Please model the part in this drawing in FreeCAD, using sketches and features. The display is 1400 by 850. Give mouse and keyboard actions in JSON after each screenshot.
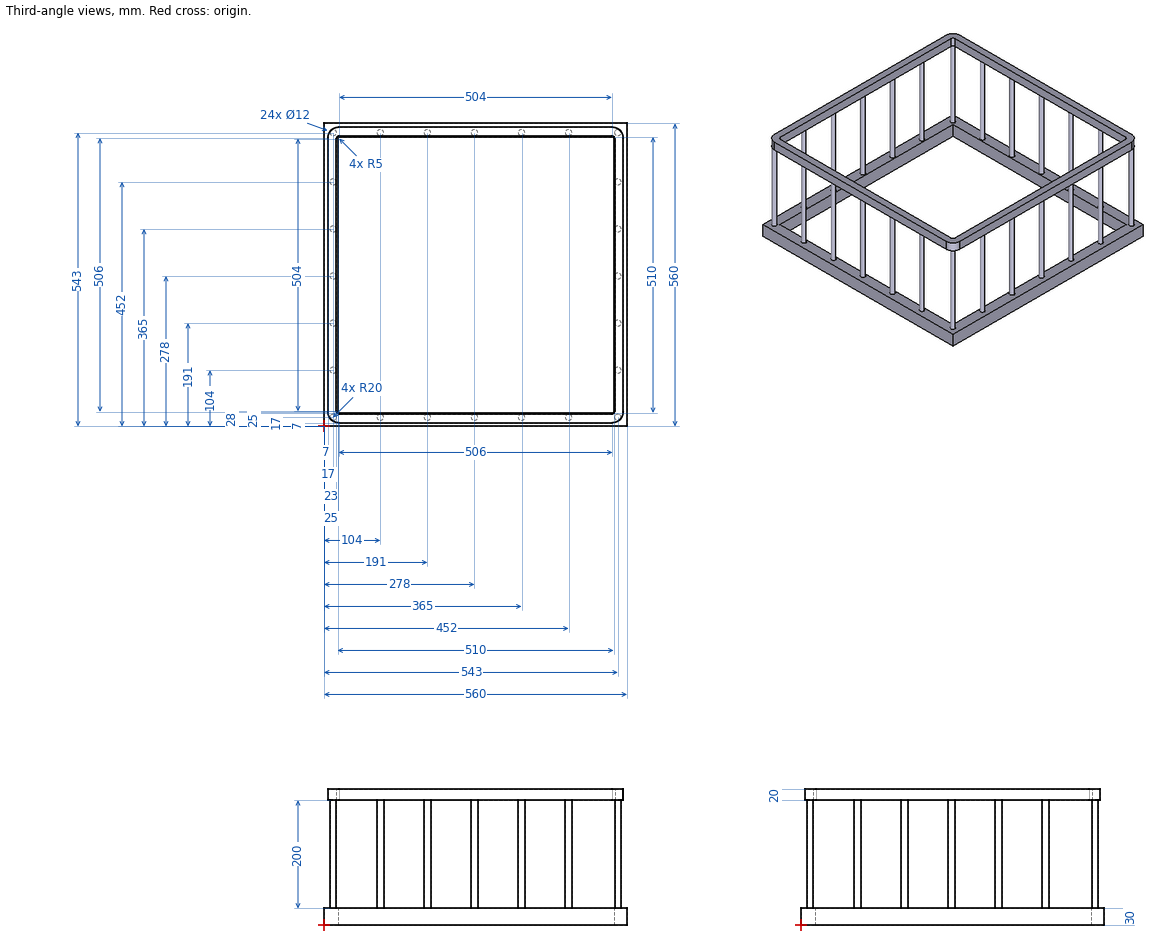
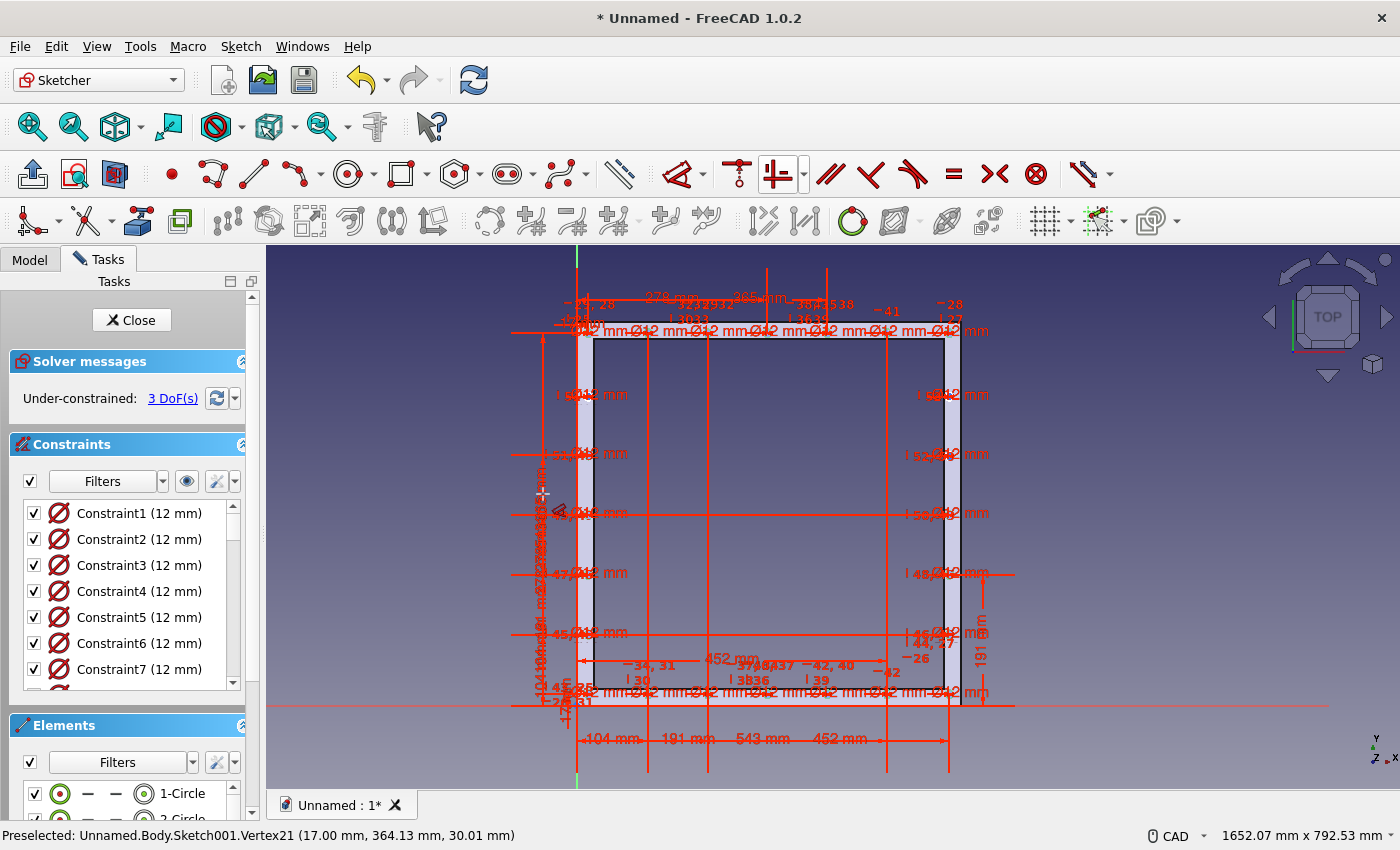
{"action": "left_click", "coordinate": [949, 456]}
{"action": "left_click", "coordinate": [983, 581]}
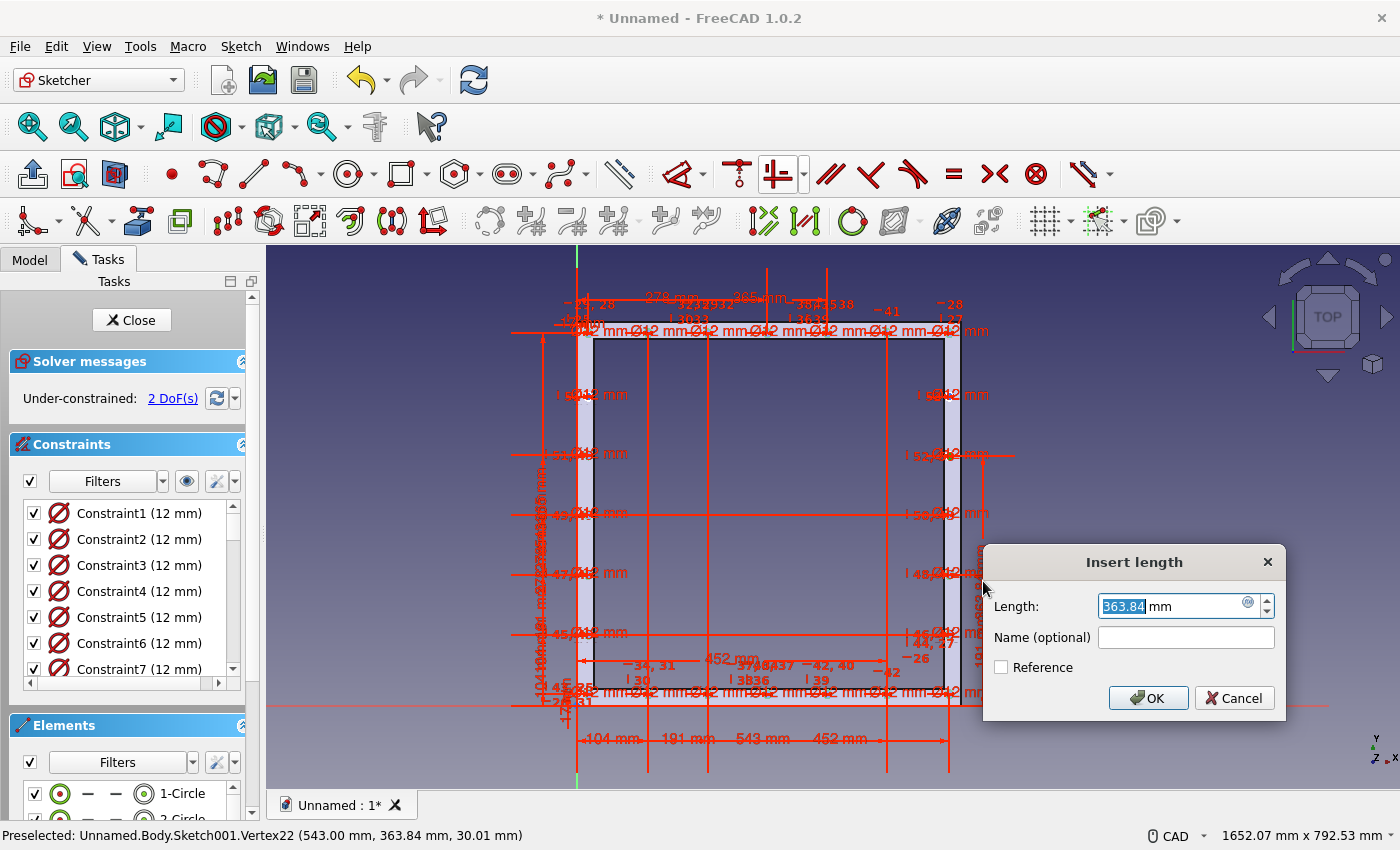
{"action": "type", "text": "365"}
{"action": "key", "text": "Return"}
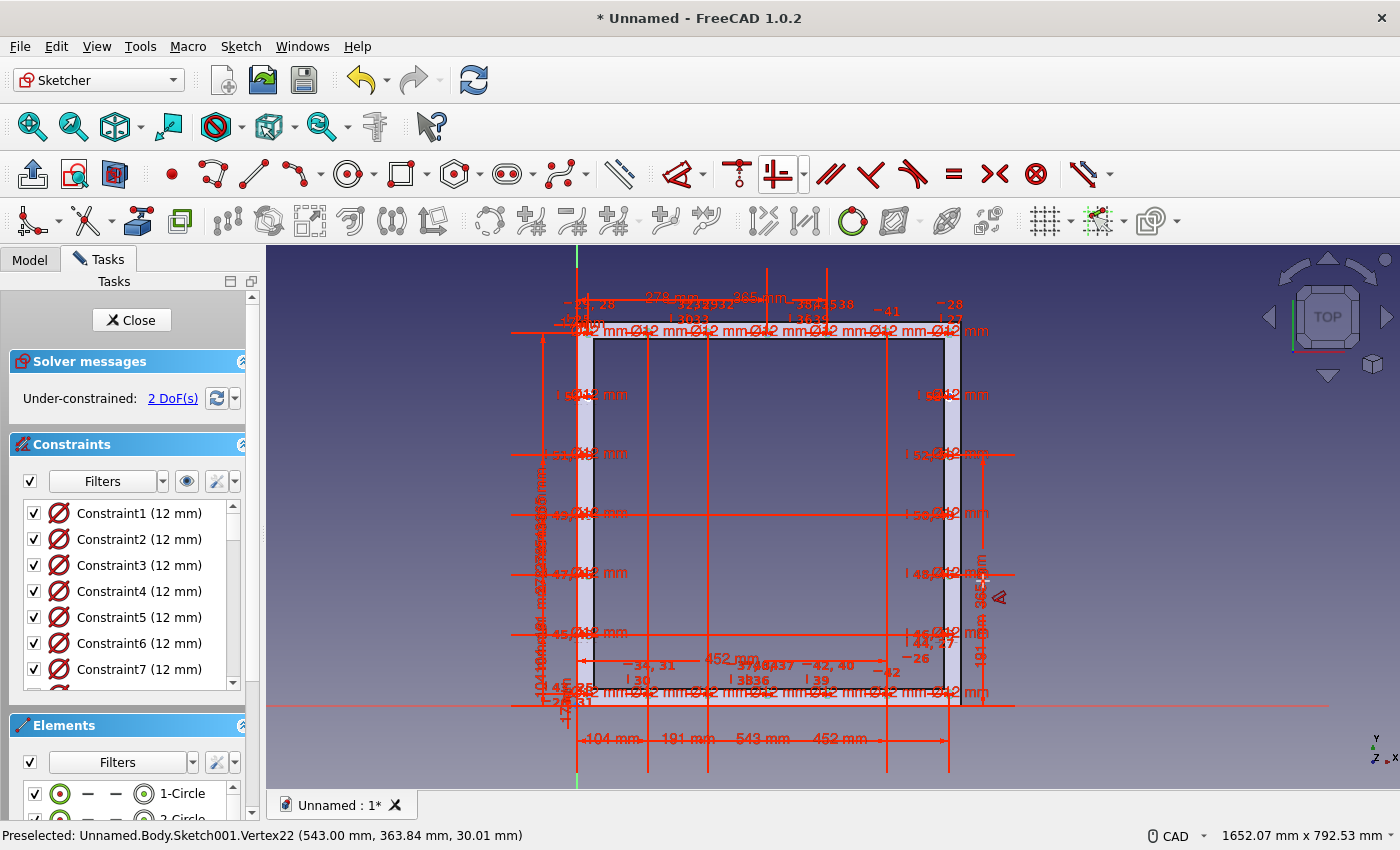
{"action": "left_click", "coordinate": [588, 397]}
{"action": "left_click", "coordinate": [543, 443]}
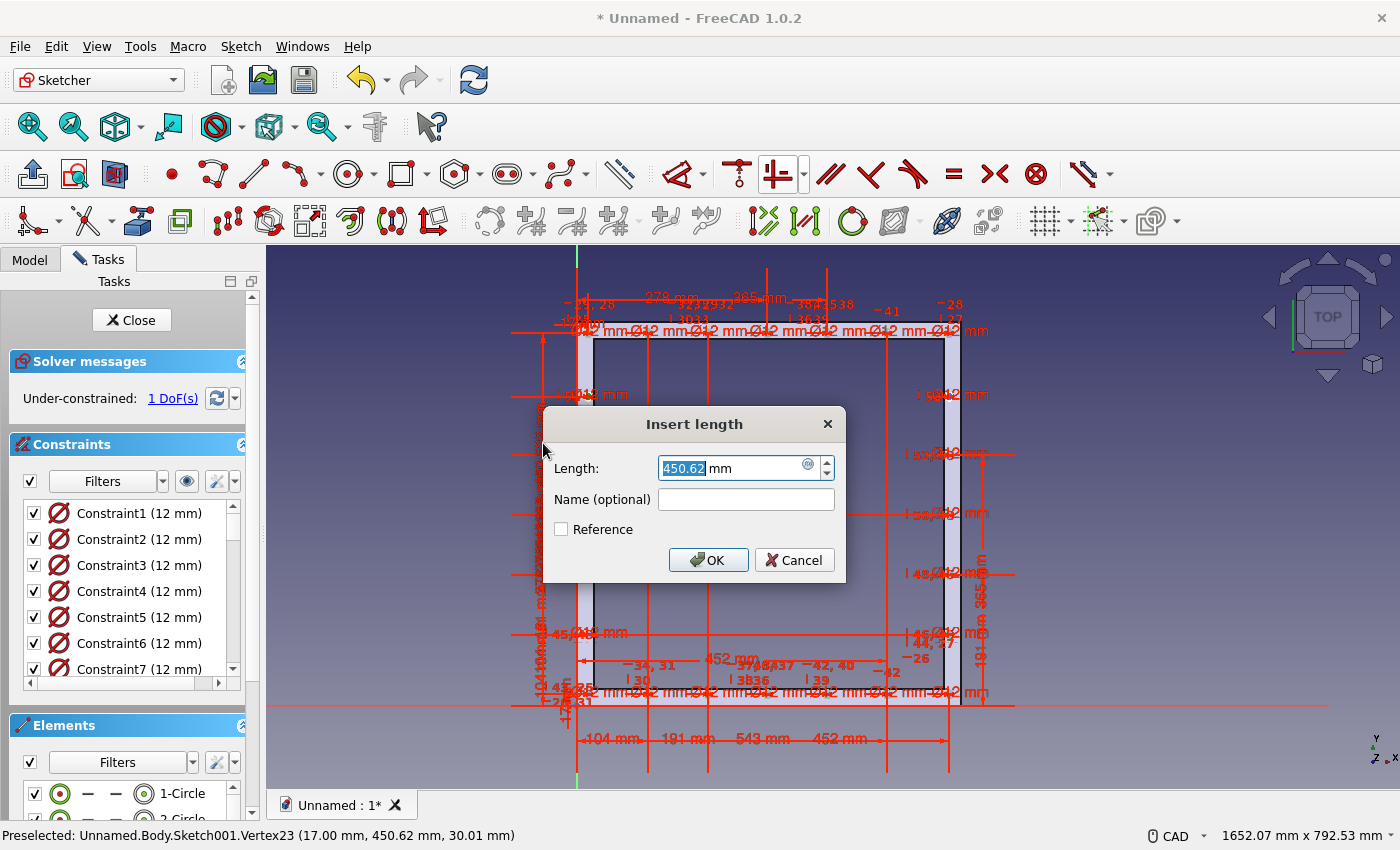
{"action": "type", "text": "452"}
{"action": "key", "text": "Return"}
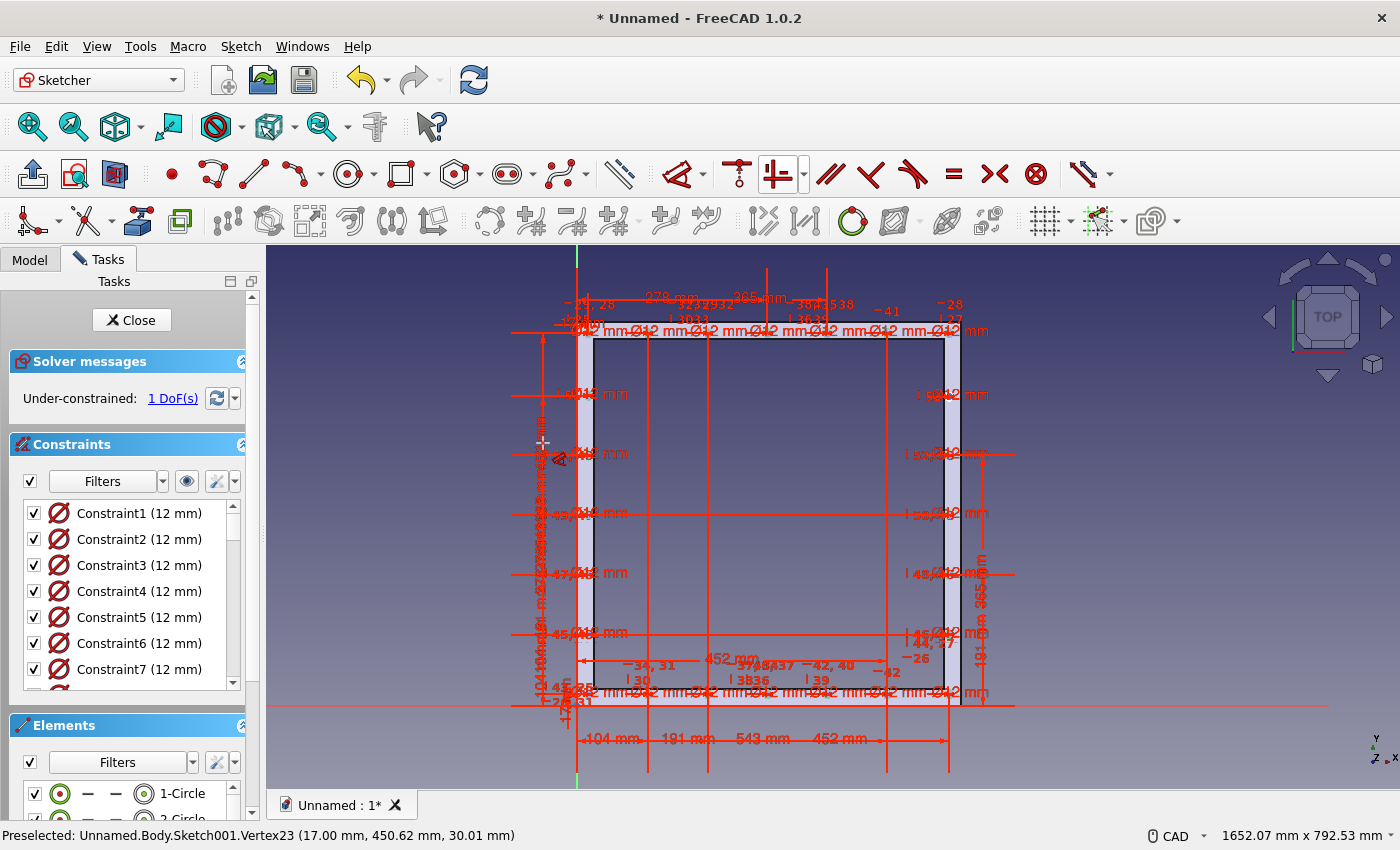
{"action": "left_click", "coordinate": [949, 397]}
{"action": "left_click", "coordinate": [983, 551]}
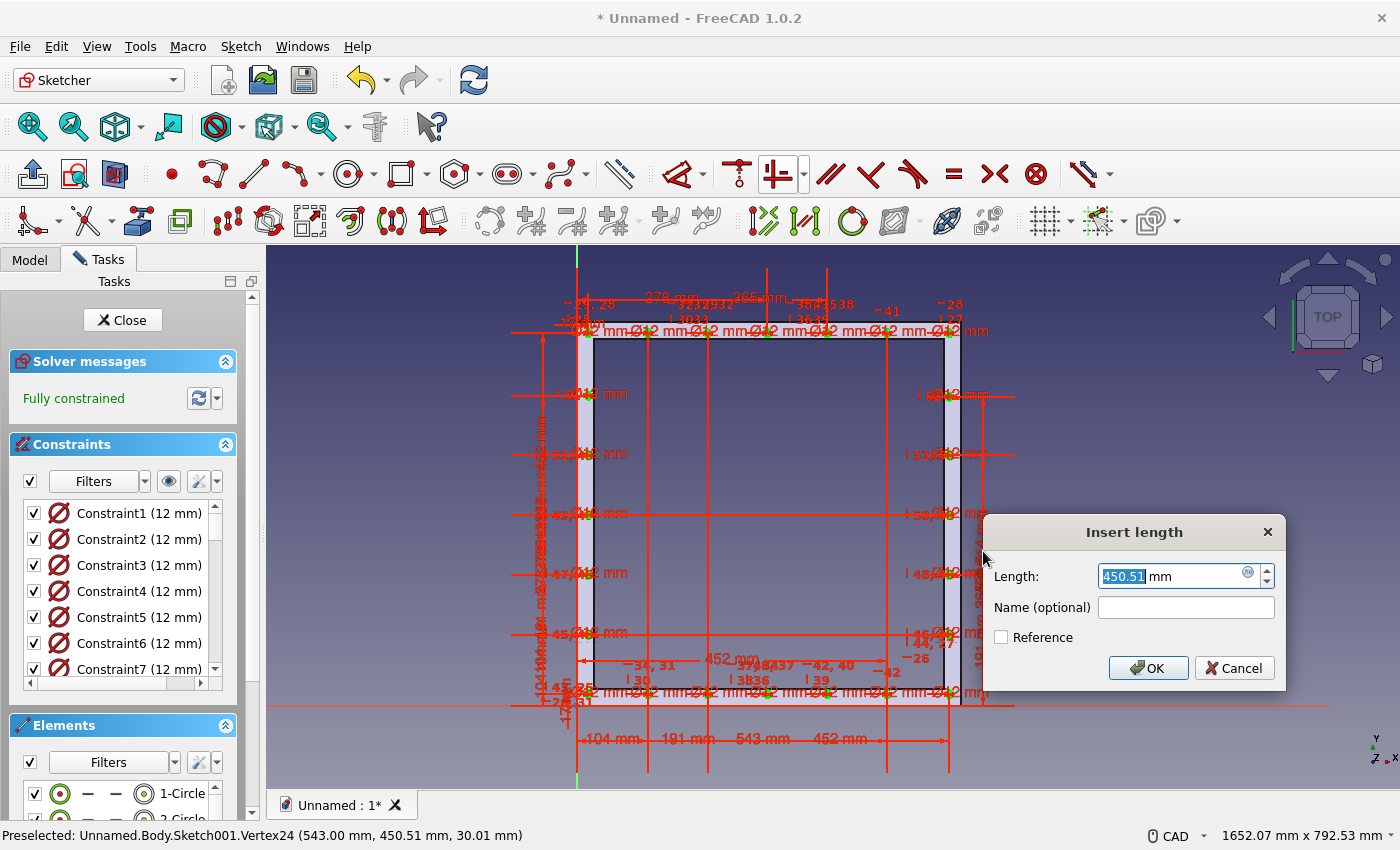
{"action": "type", "text": "452"}
{"action": "key", "text": "Return"}
{"action": "key", "text": "Escape"}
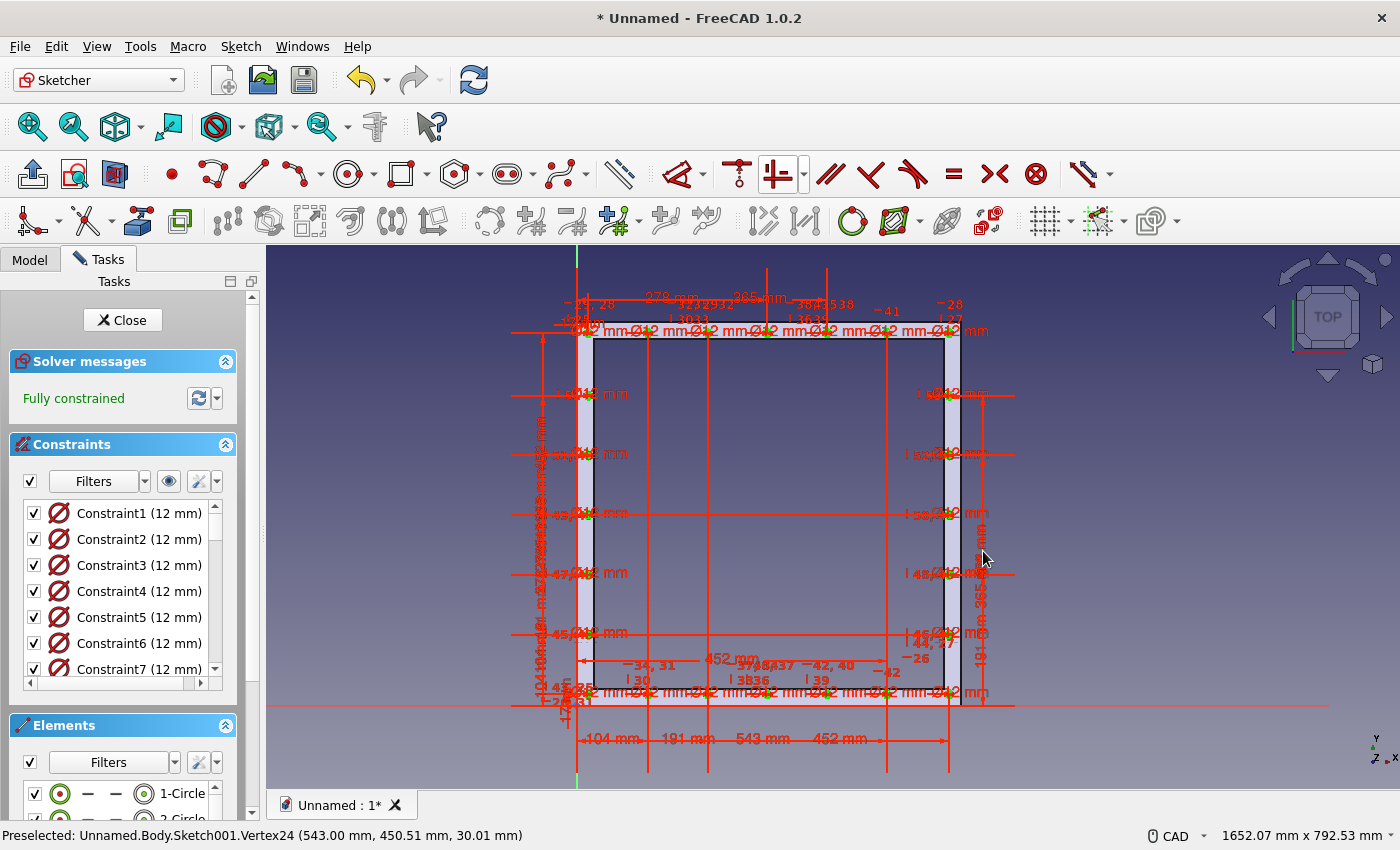
{"action": "left_click", "coordinate": [123, 320]}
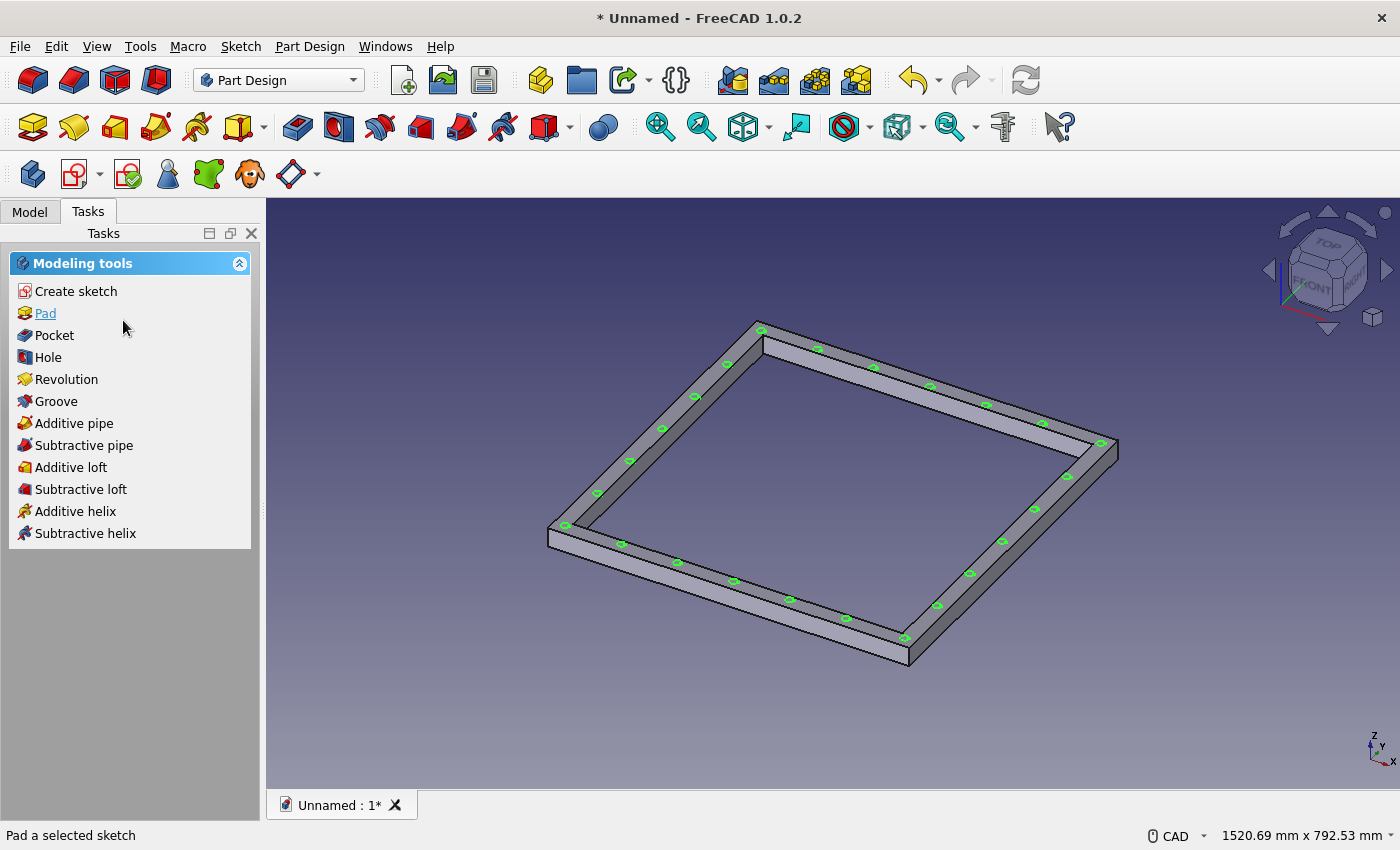
{"action": "left_click", "coordinate": [33, 128]}